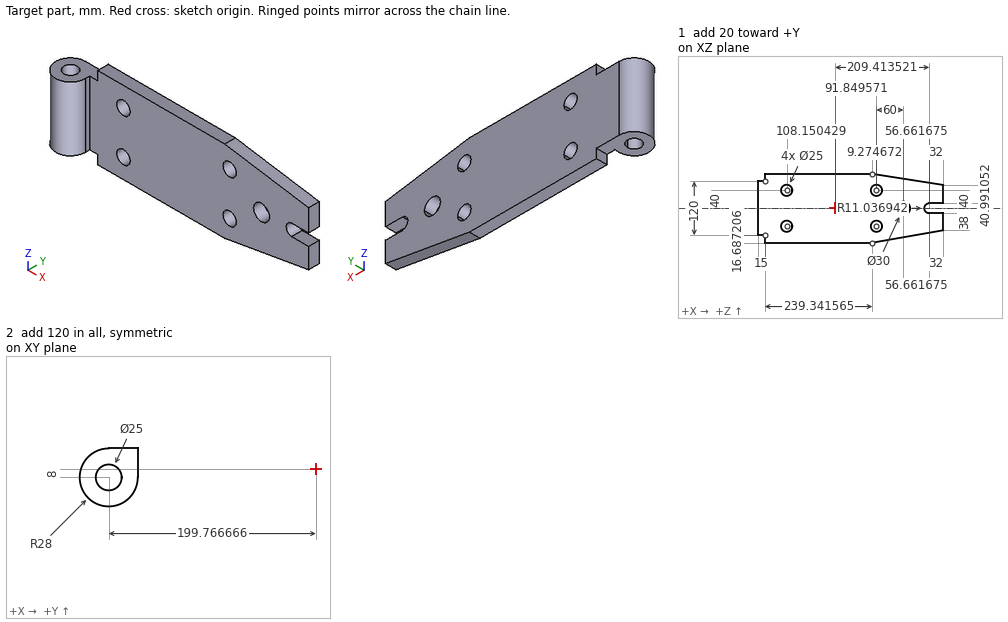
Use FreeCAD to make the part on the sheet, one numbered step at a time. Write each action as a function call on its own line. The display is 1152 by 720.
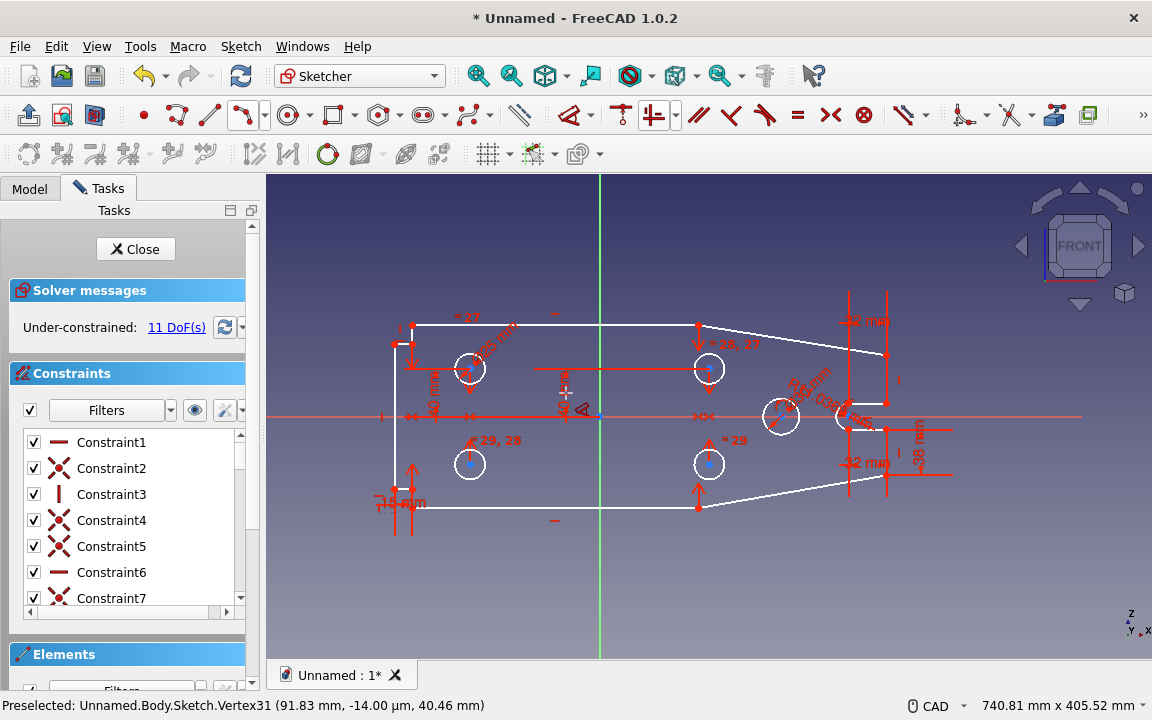
click(395, 446)
click(361, 383)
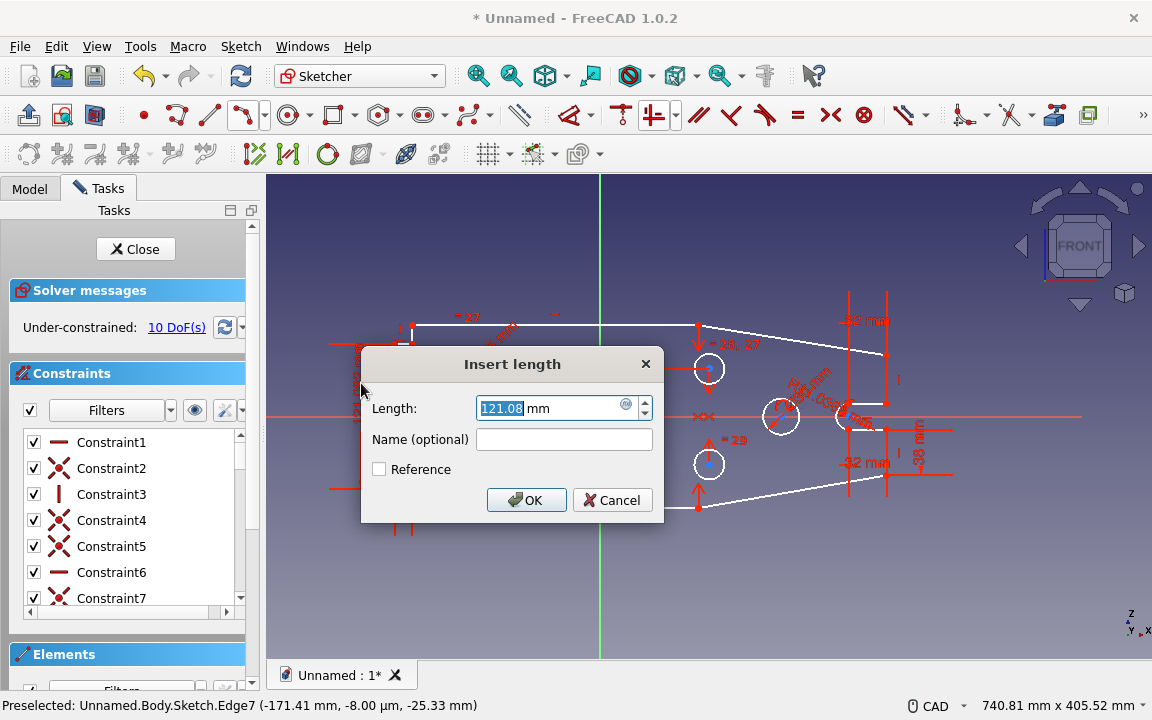
text(120)
key(Return)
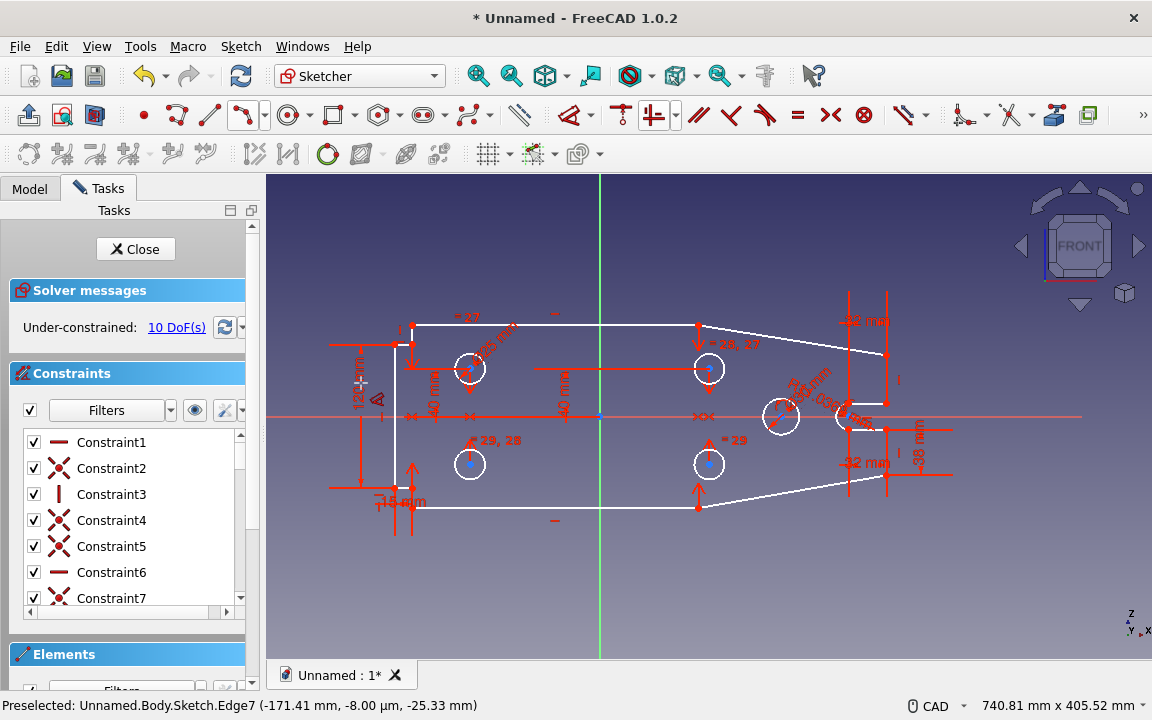
click(709, 369)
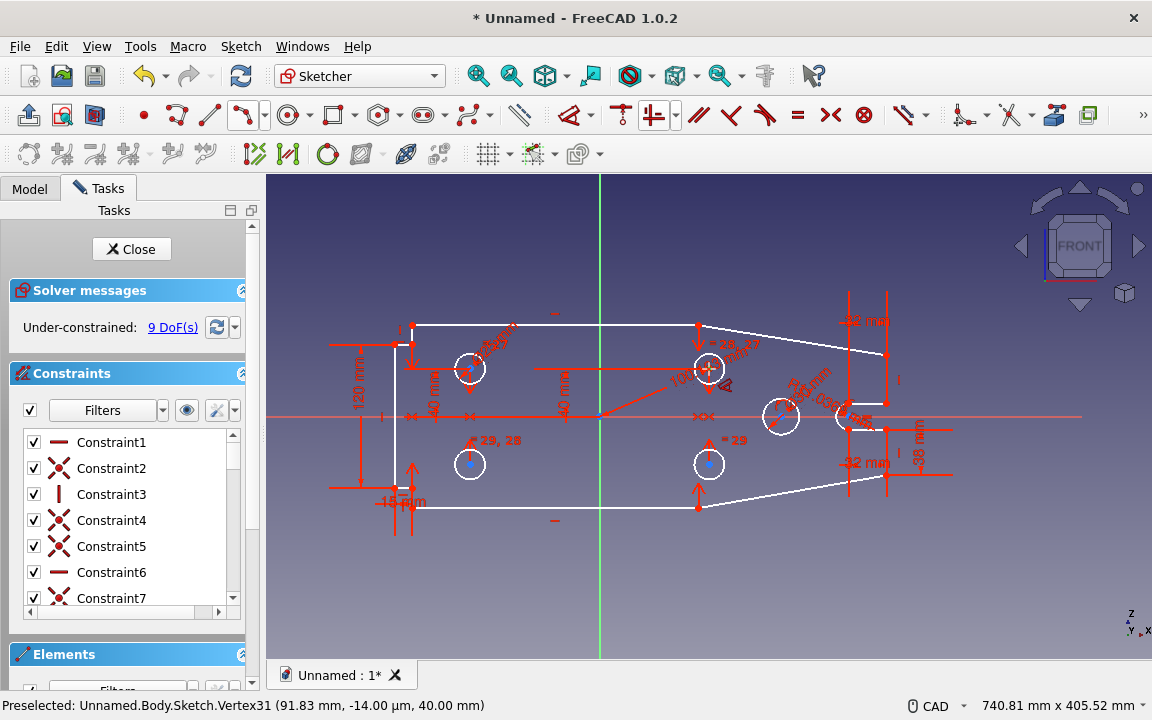
click(781, 417)
click(745, 451)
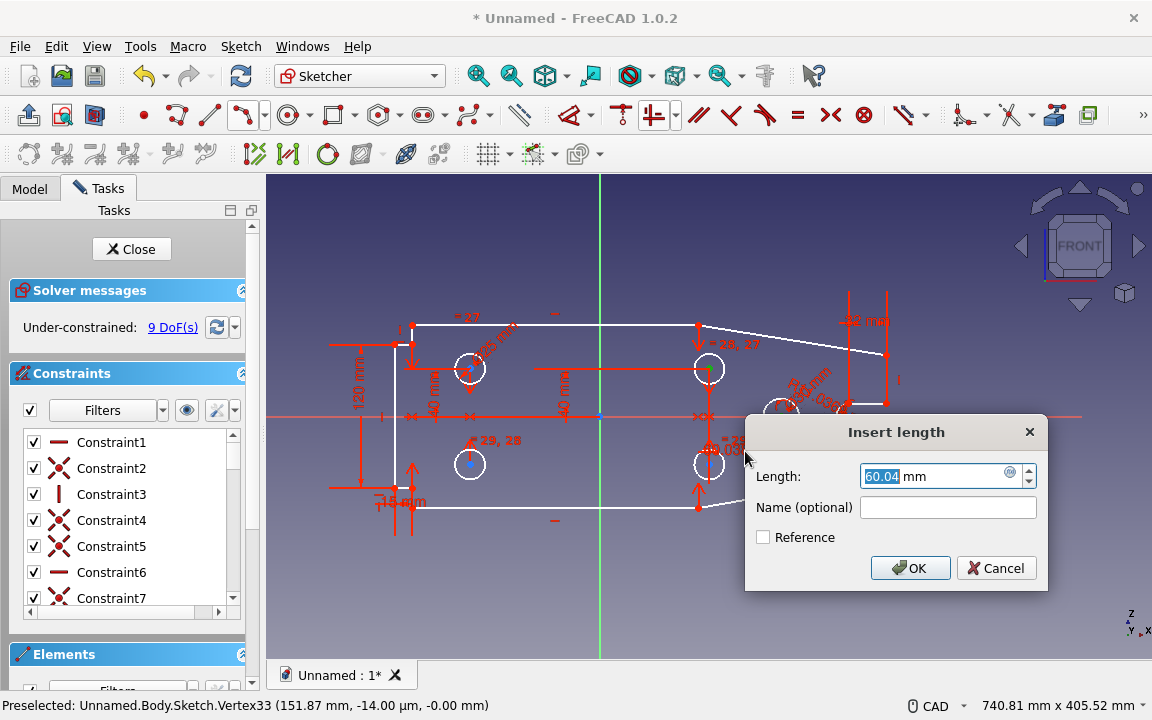
text(60)
key(Return)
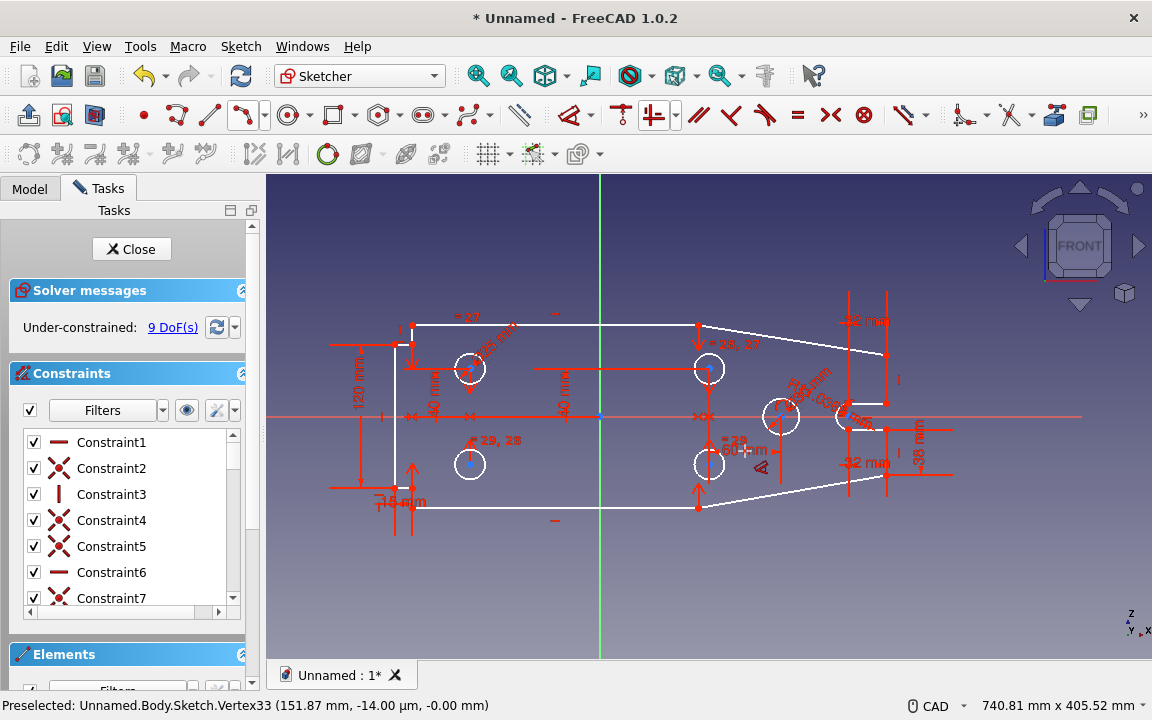
scroll(412, 498, up, 4)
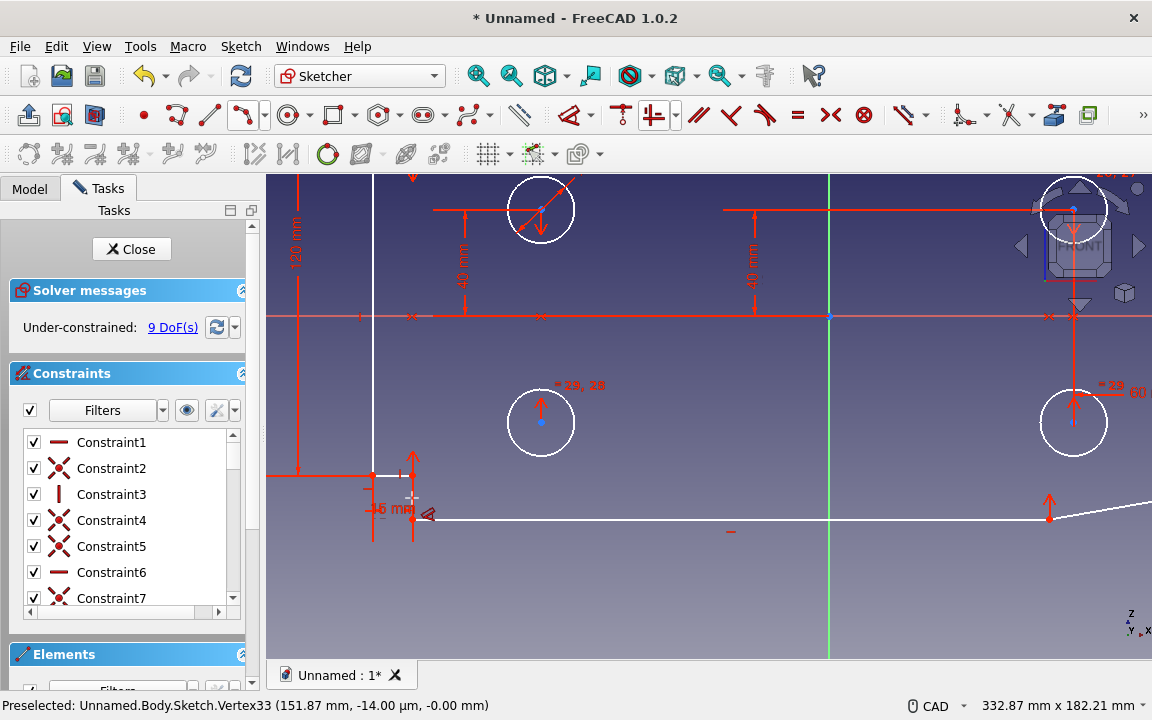
click(413, 498)
click(447, 488)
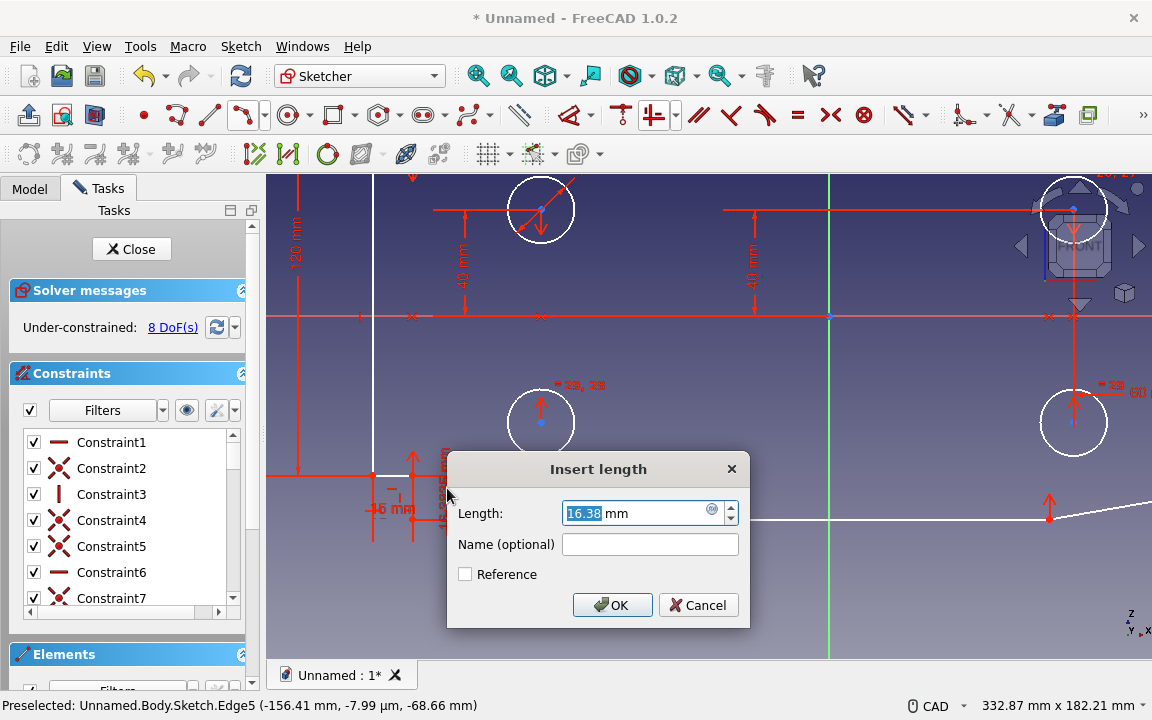
text(16.687206)
key(Return)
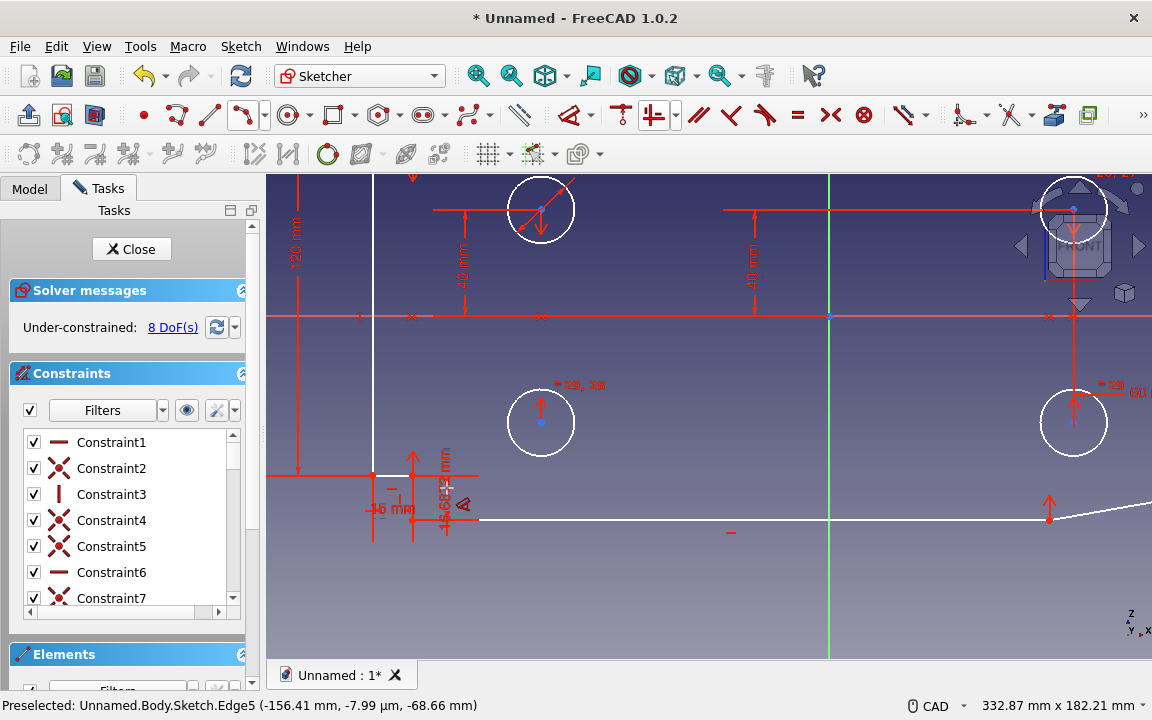
scroll(412, 498, down, 4)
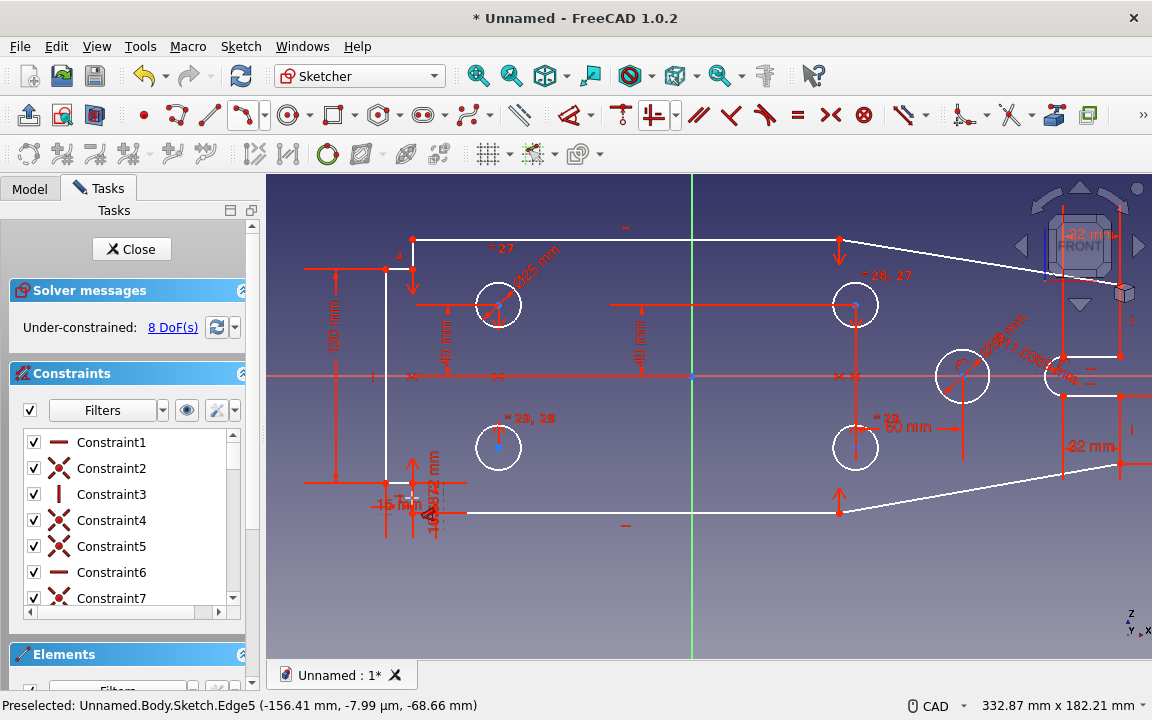
click(887, 370)
click(921, 379)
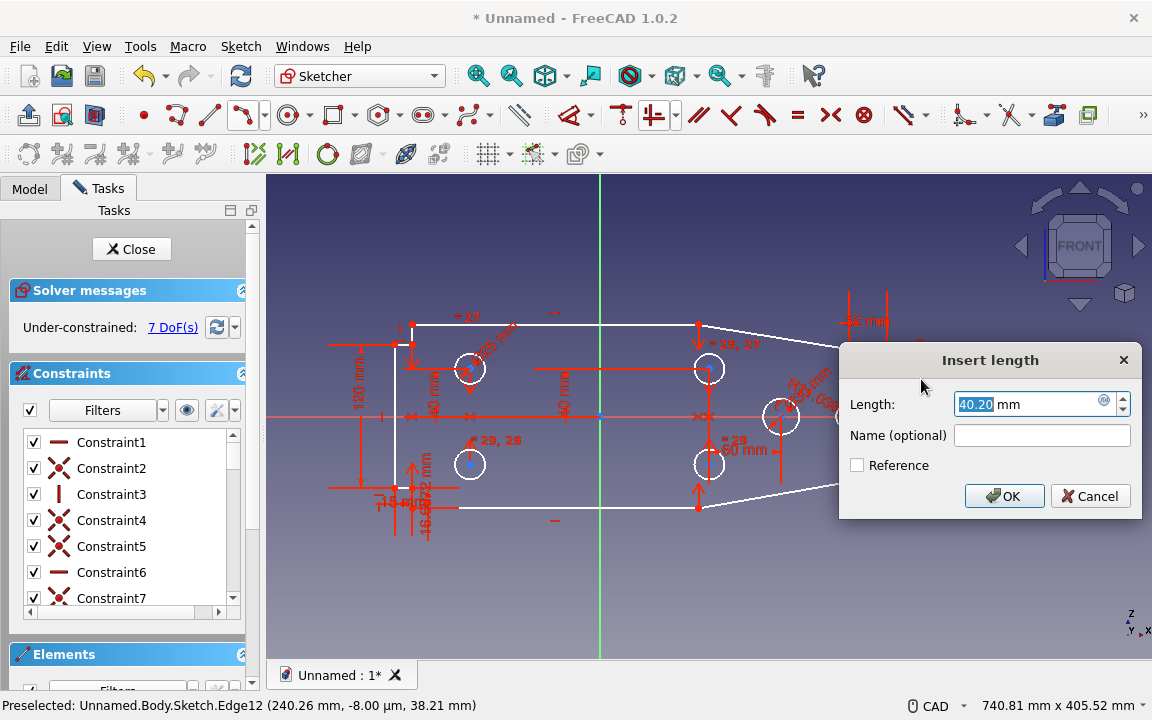
text(40.991052)
key(Return)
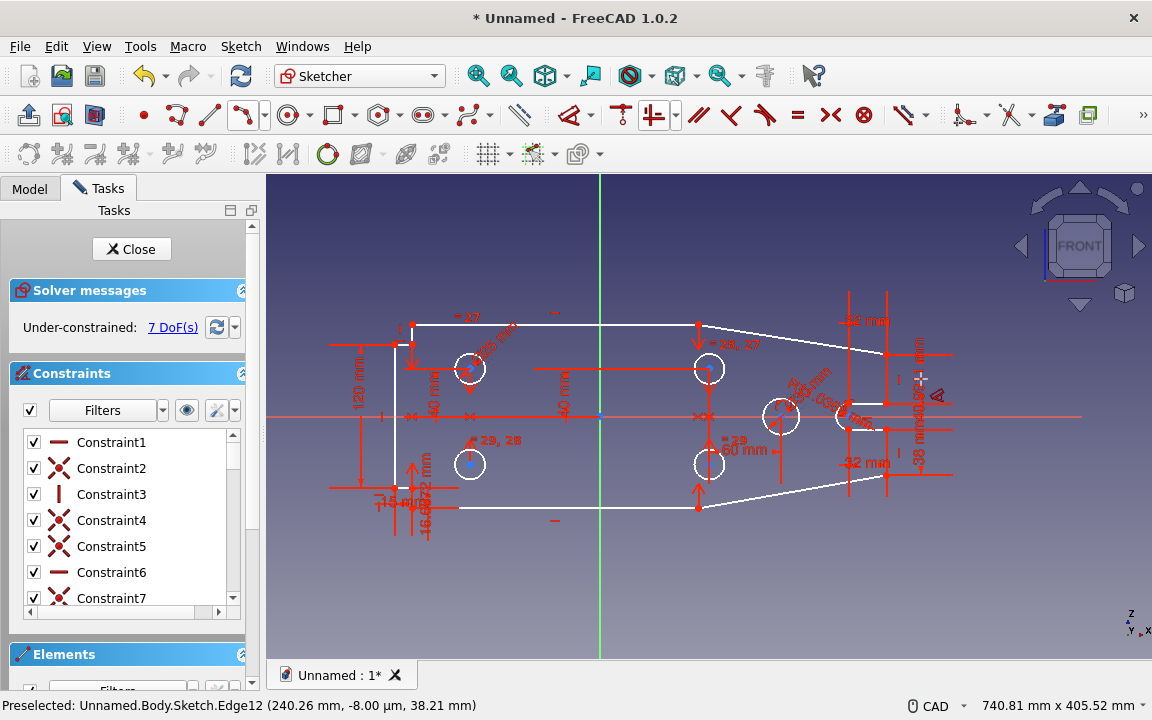
click(709, 369)
click(654, 451)